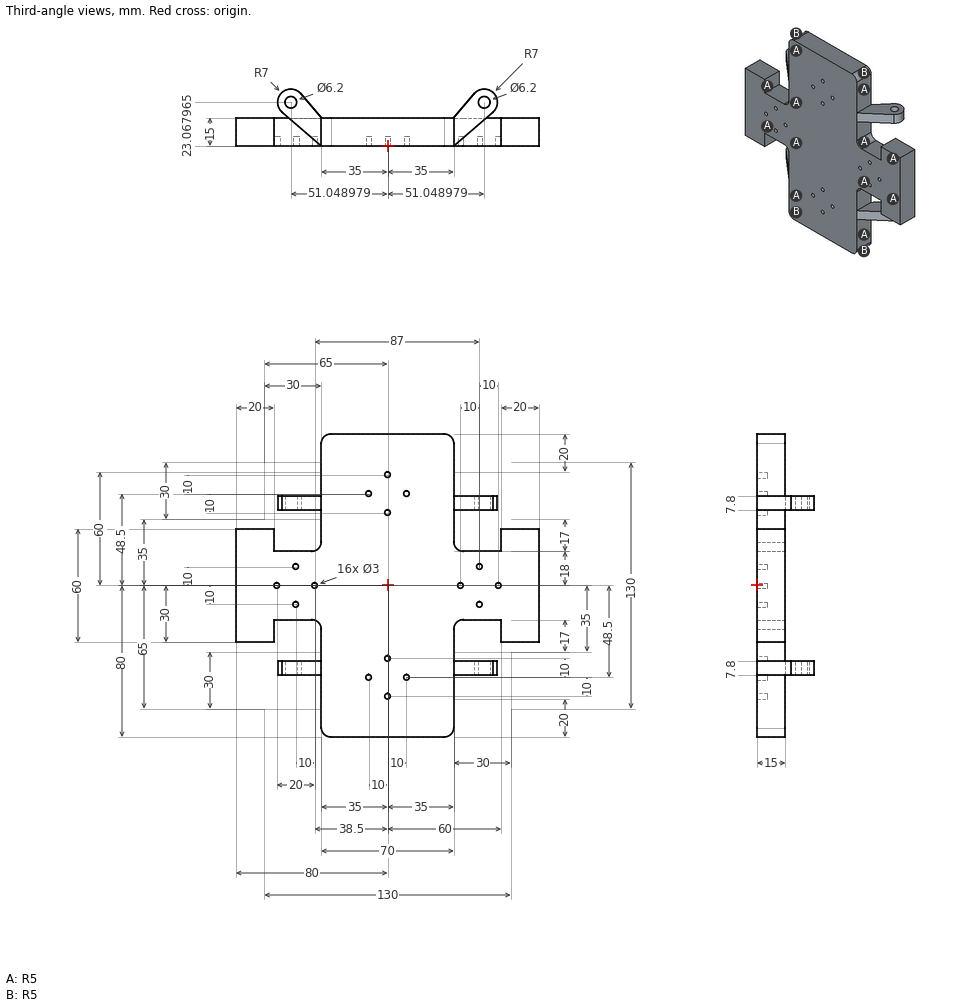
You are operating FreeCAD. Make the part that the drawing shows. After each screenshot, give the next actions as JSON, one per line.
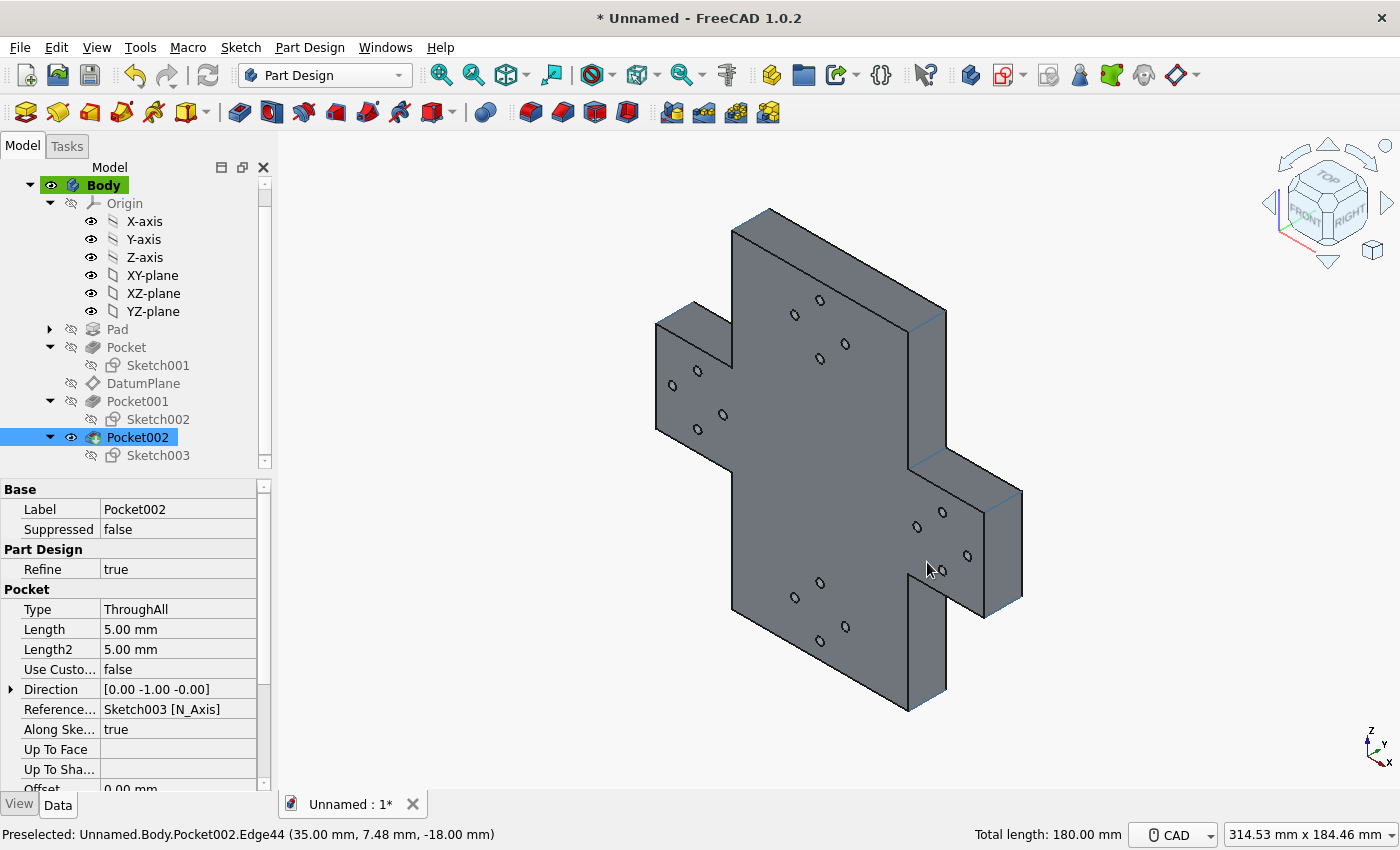
{"action": "left_click", "coordinate": [532, 112]}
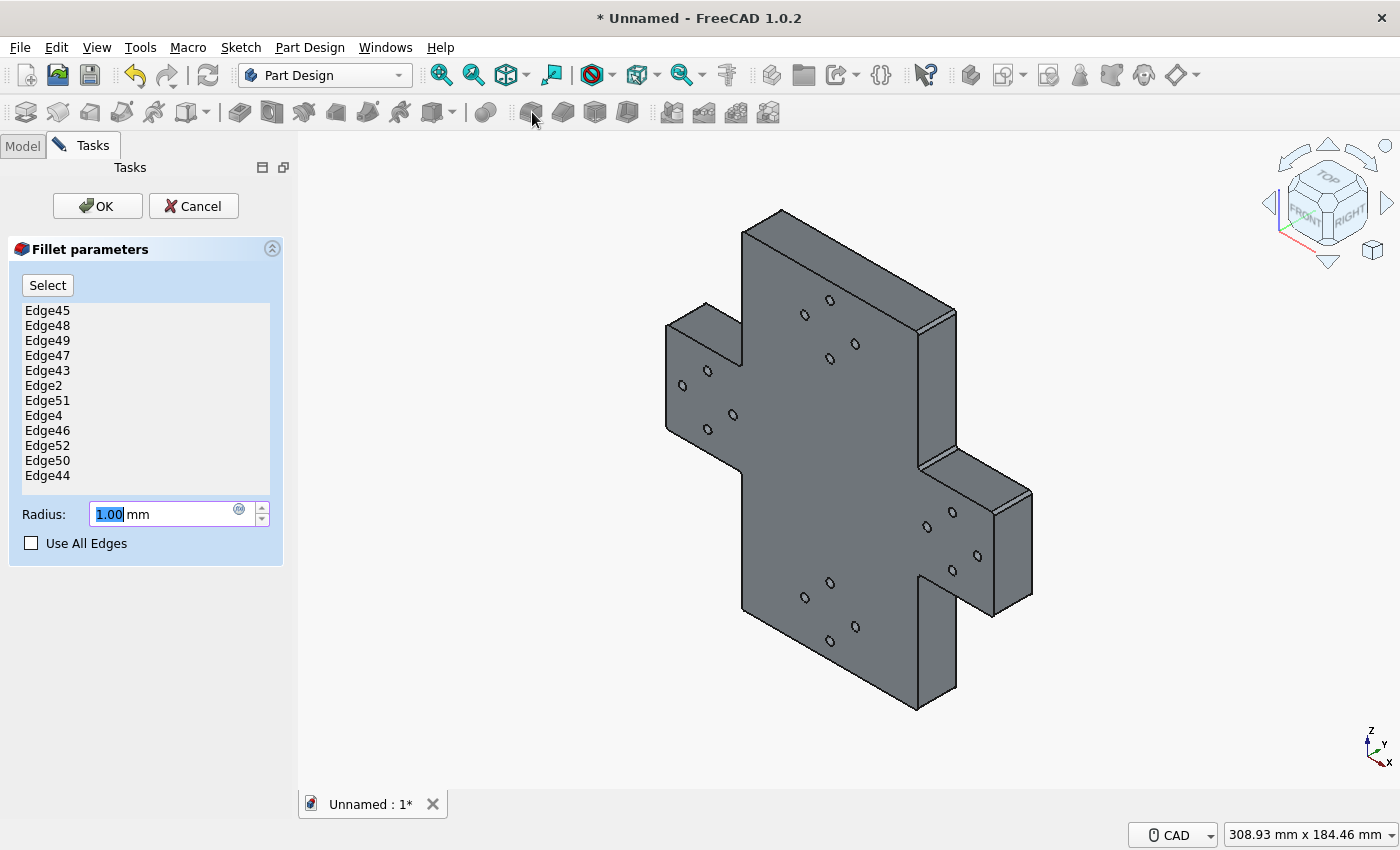
{"action": "type", "text": "5"}
{"action": "key", "text": "Tab"}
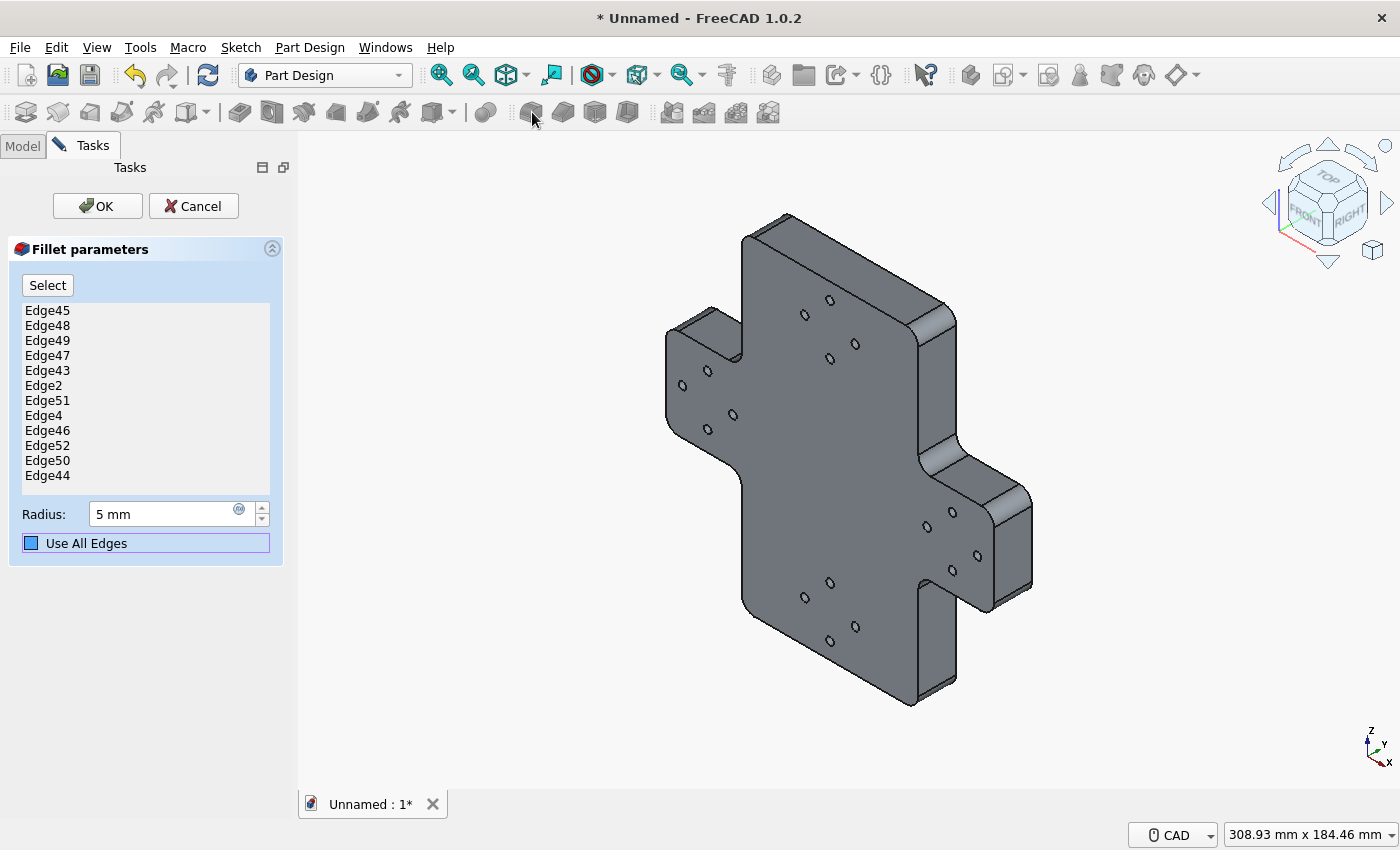
{"action": "left_click", "coordinate": [98, 206]}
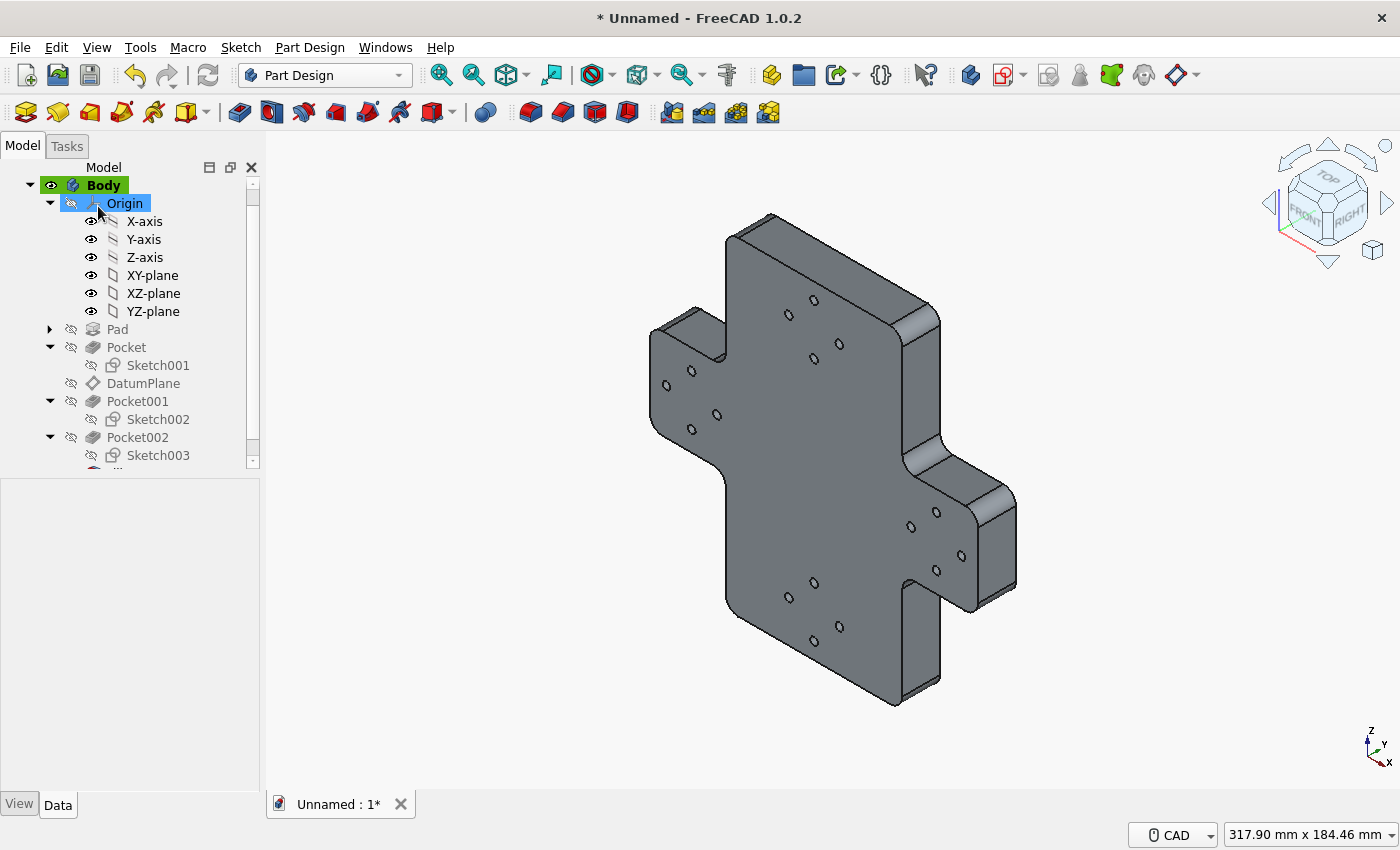
{"action": "key", "text": "4"}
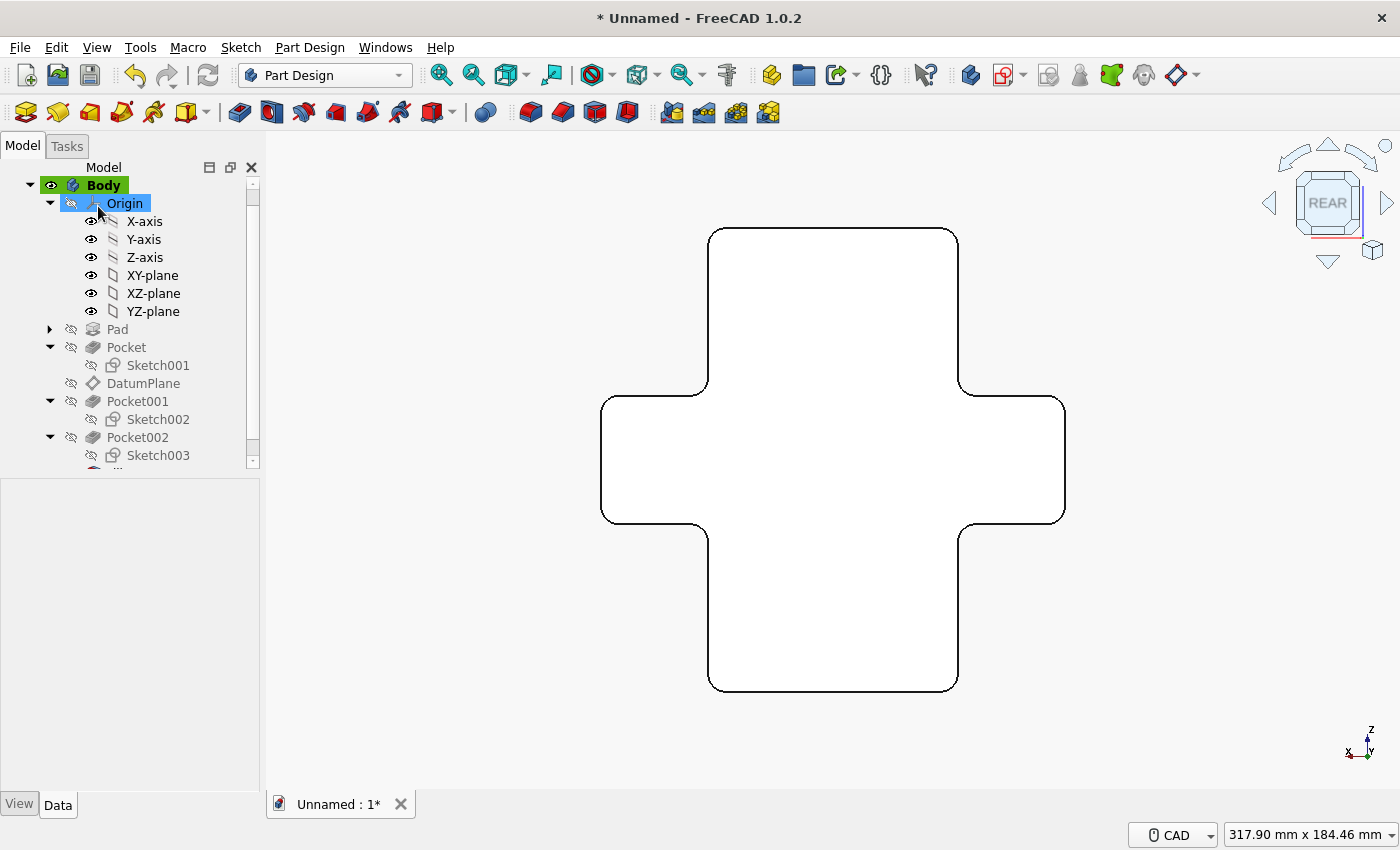
{"action": "left_click", "coordinate": [833, 459]}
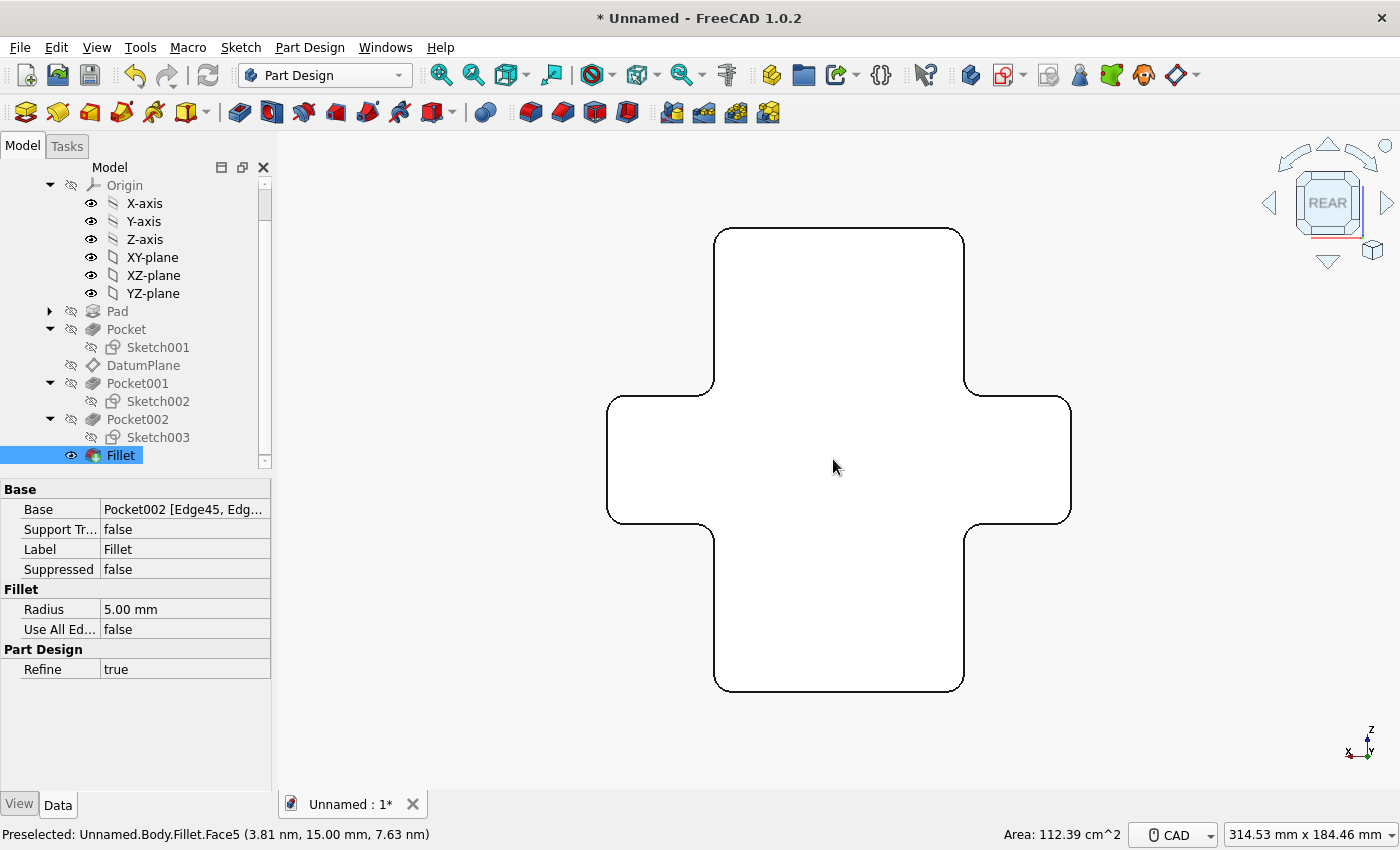
{"action": "left_click", "coordinate": [1004, 76]}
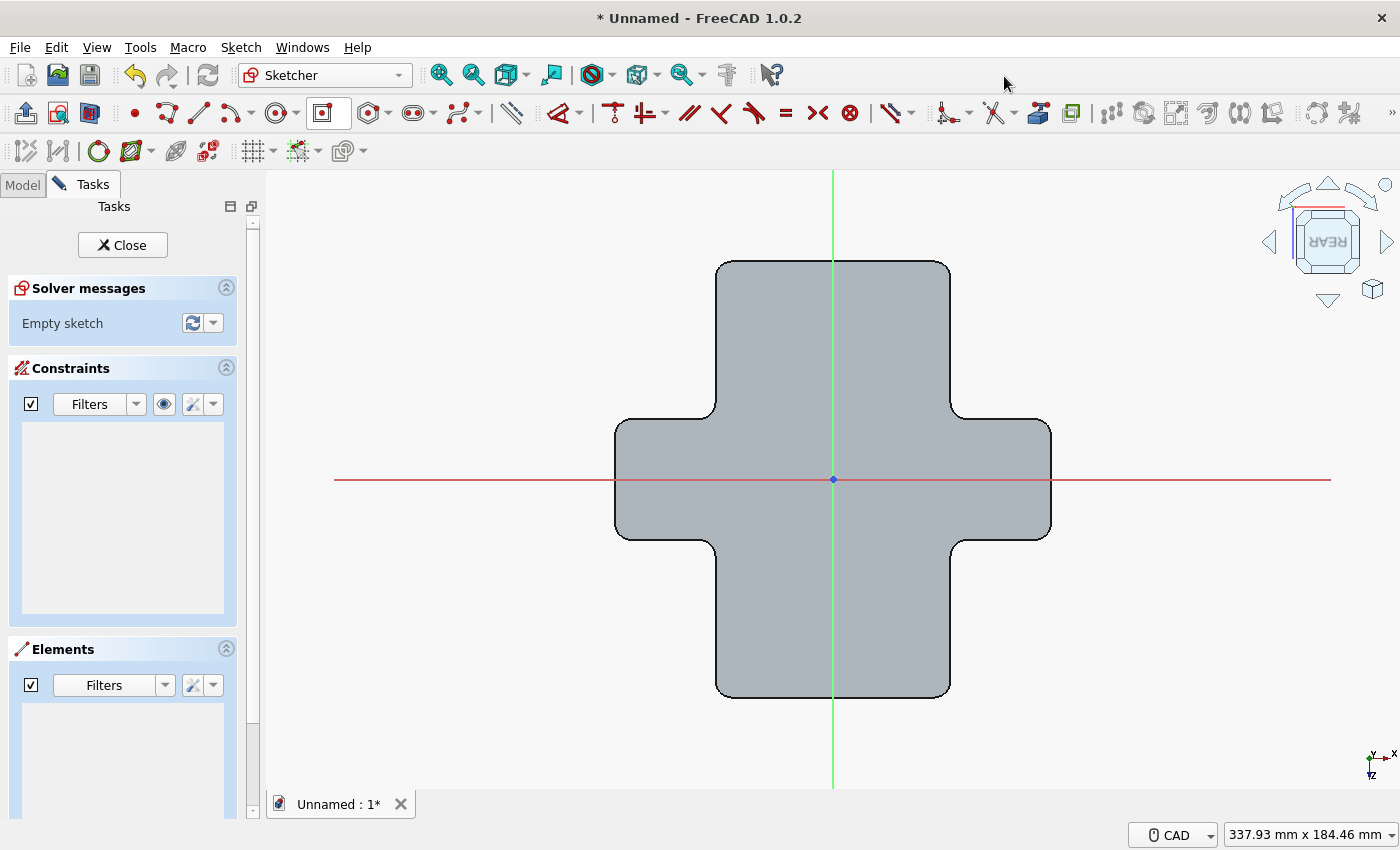
{"action": "scroll", "coordinate": [625, 480], "scroll_direction": "down", "scroll_amount": 2}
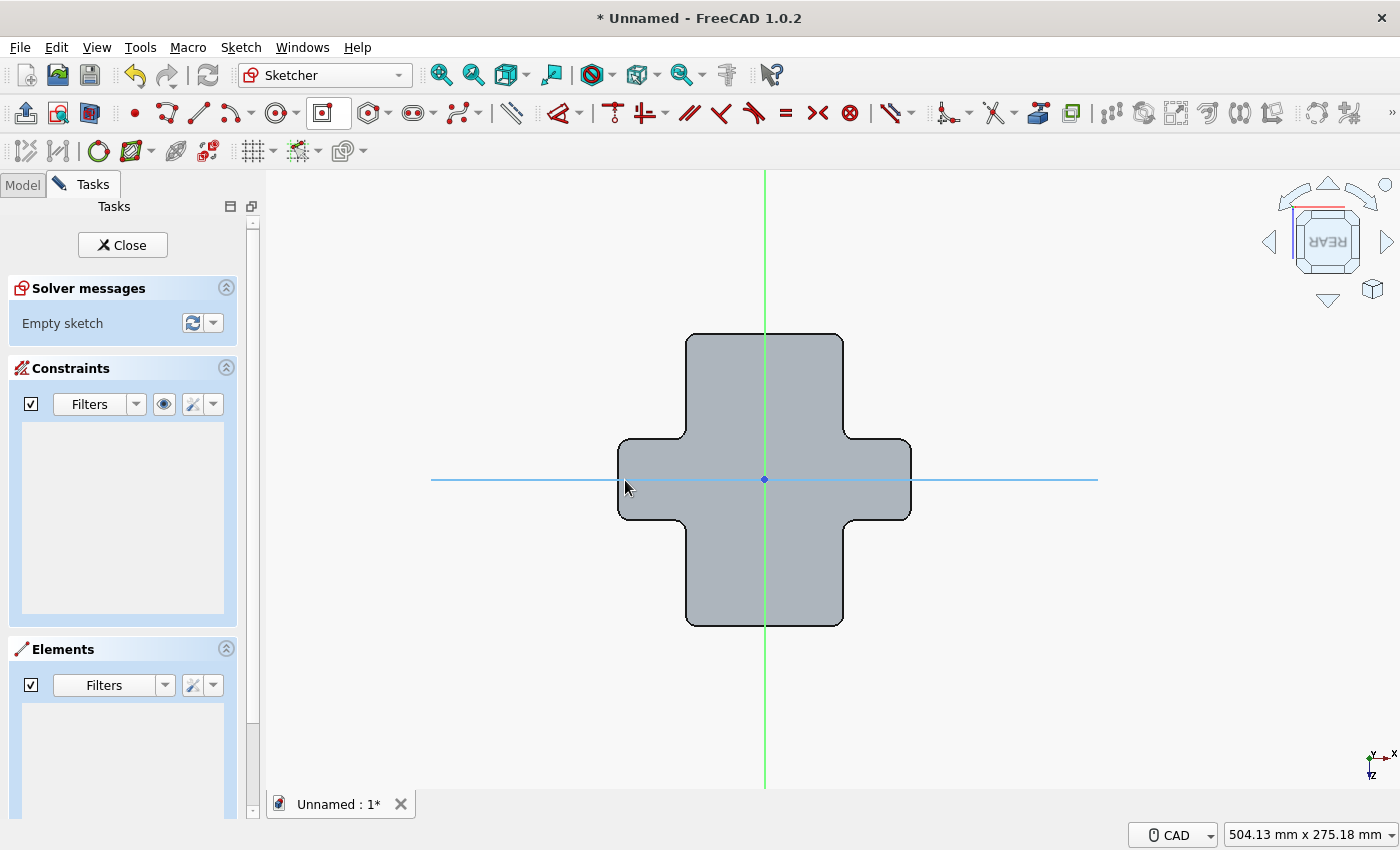
{"action": "key", "text": "g r"}